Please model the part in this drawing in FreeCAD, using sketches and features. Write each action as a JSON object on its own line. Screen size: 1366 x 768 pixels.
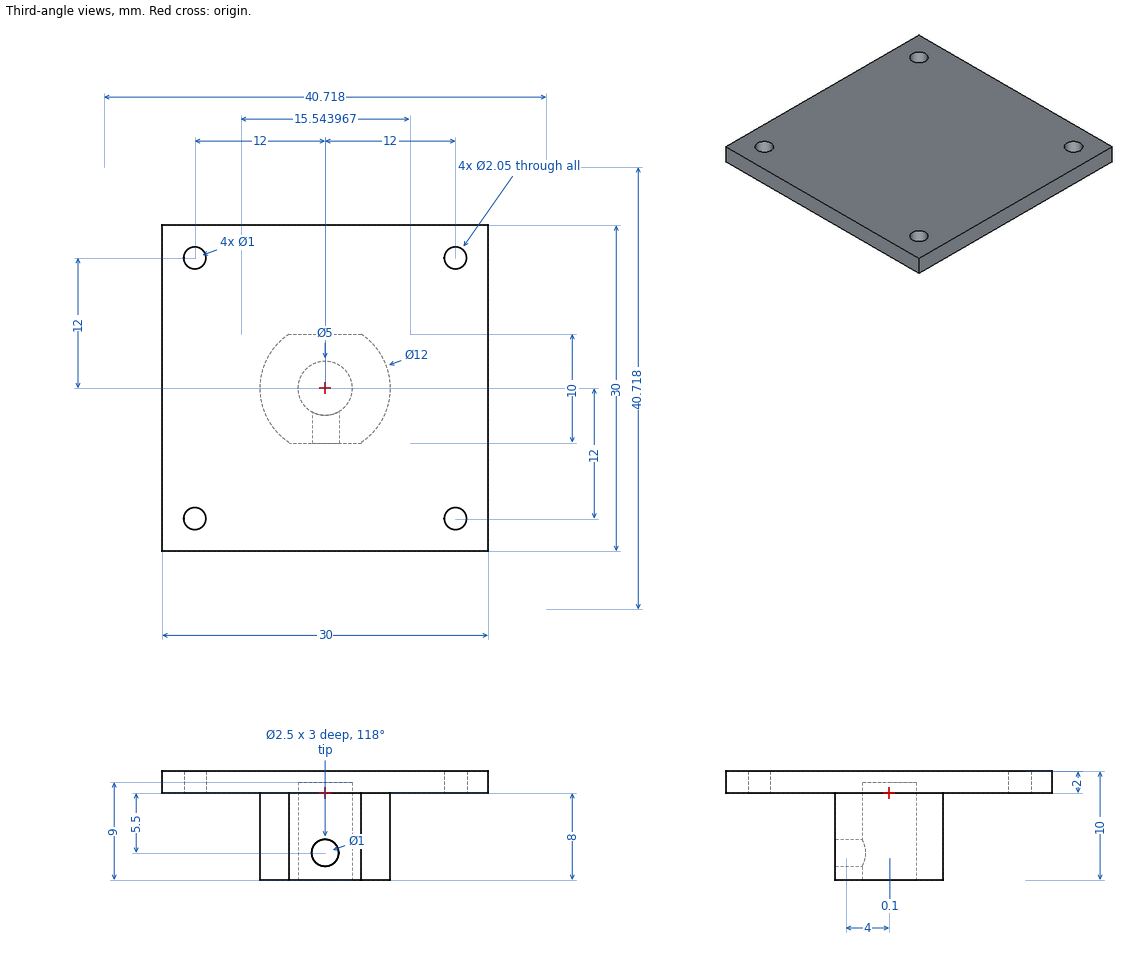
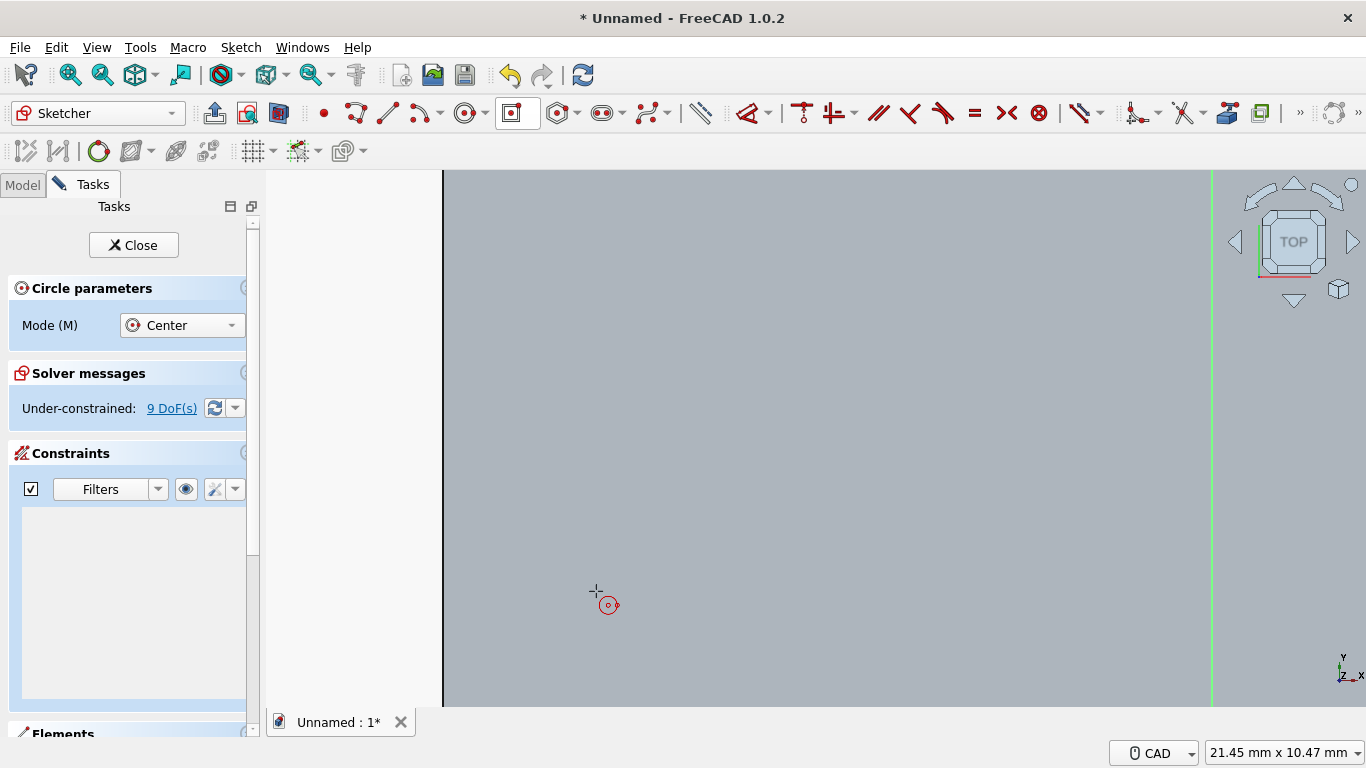
{"action": "scroll", "coordinate": [595, 591], "scroll_direction": "down", "scroll_amount": 7}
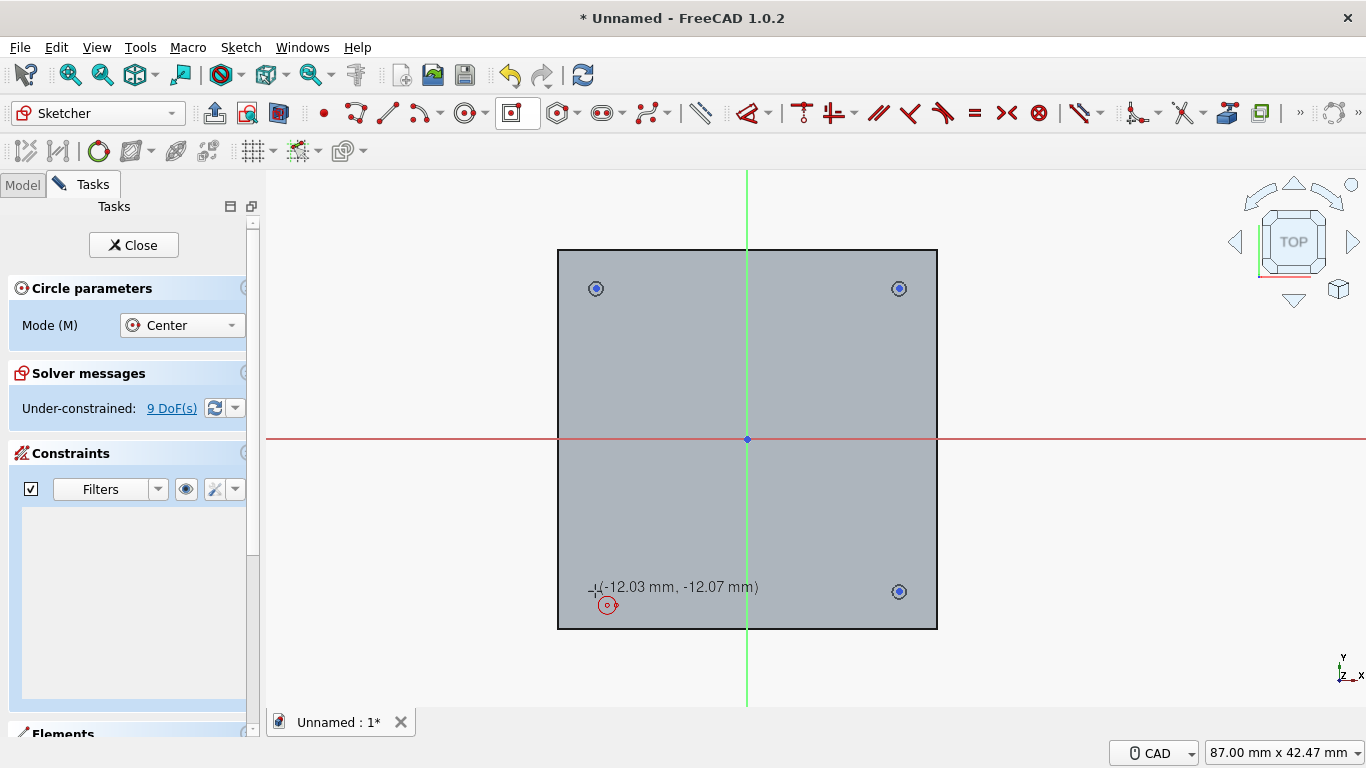
{"action": "left_click", "coordinate": [596, 591]}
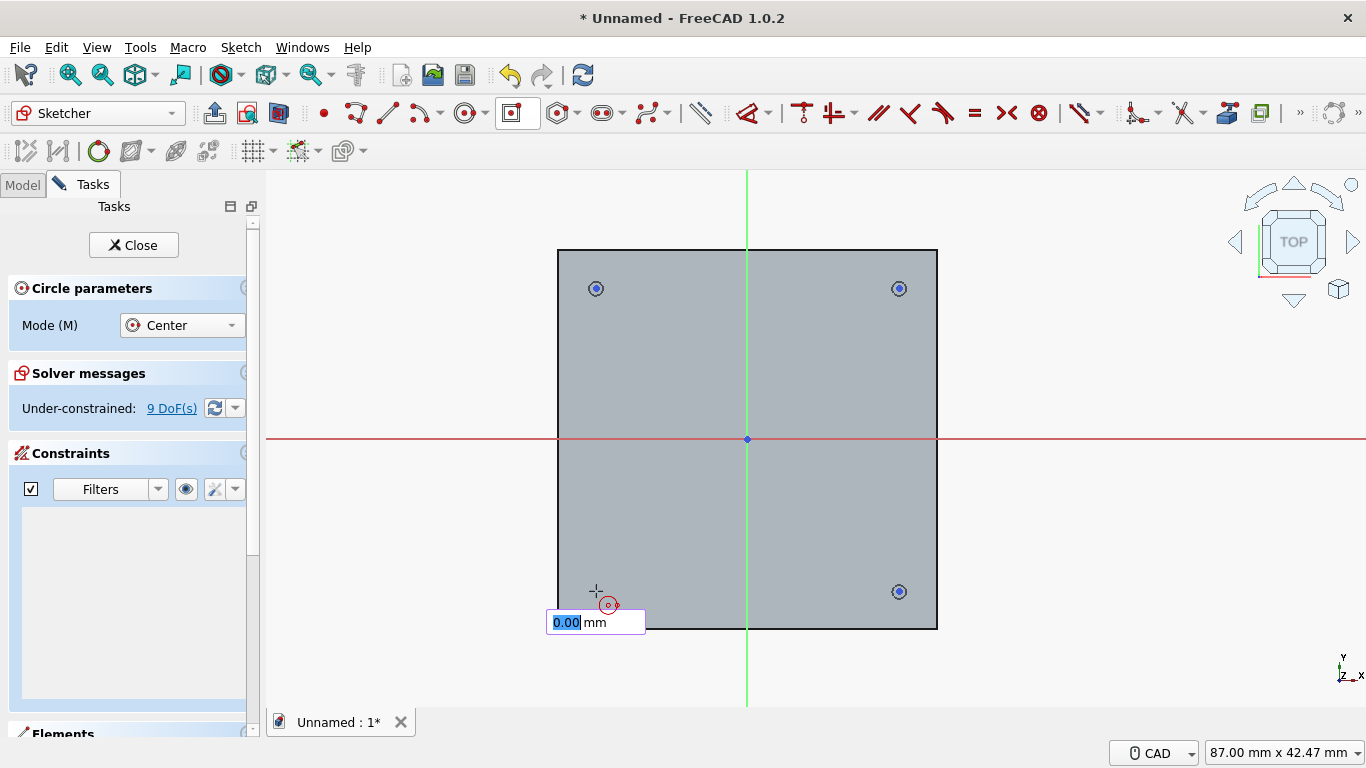
{"action": "scroll", "coordinate": [600, 587], "scroll_direction": "up", "scroll_amount": 5}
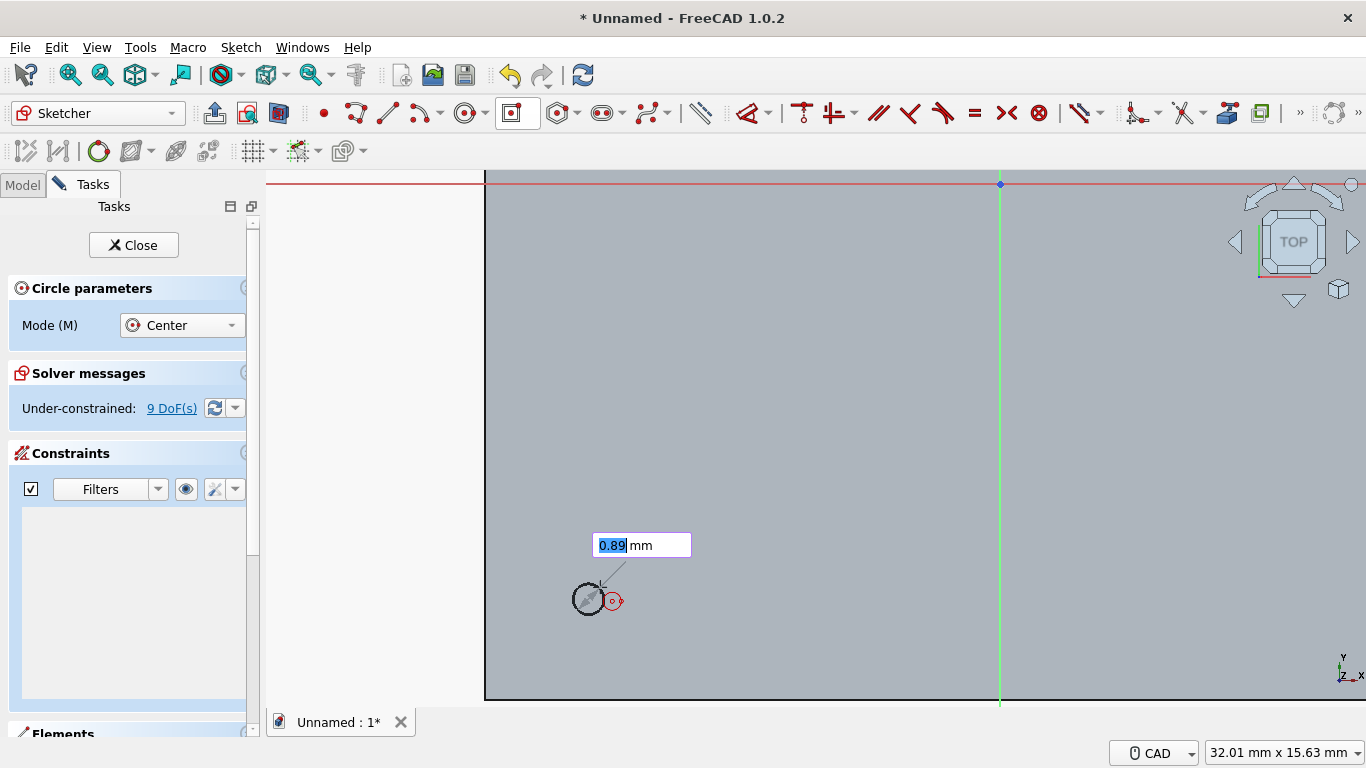
{"action": "left_click", "coordinate": [600, 584]}
{"action": "key", "text": "Escape"}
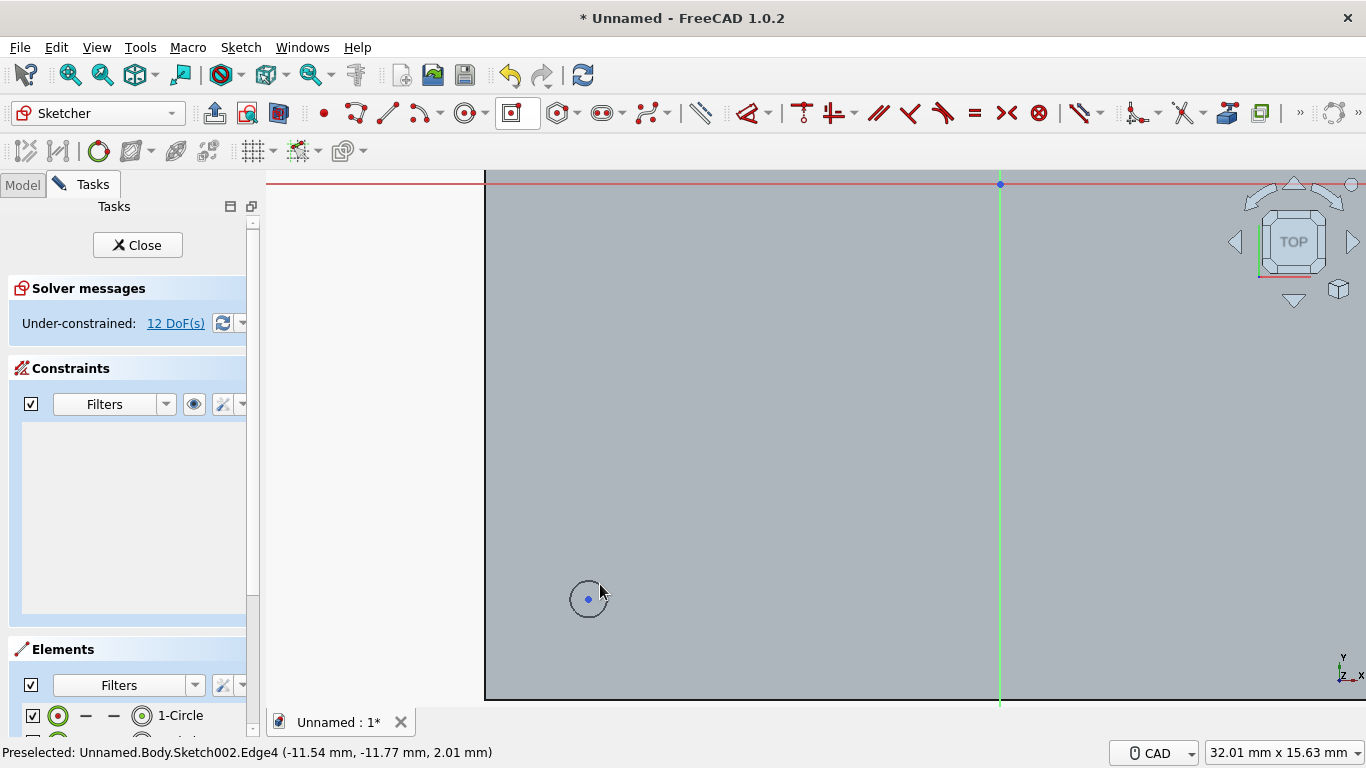
{"action": "scroll", "coordinate": [600, 587], "scroll_direction": "down", "scroll_amount": 5}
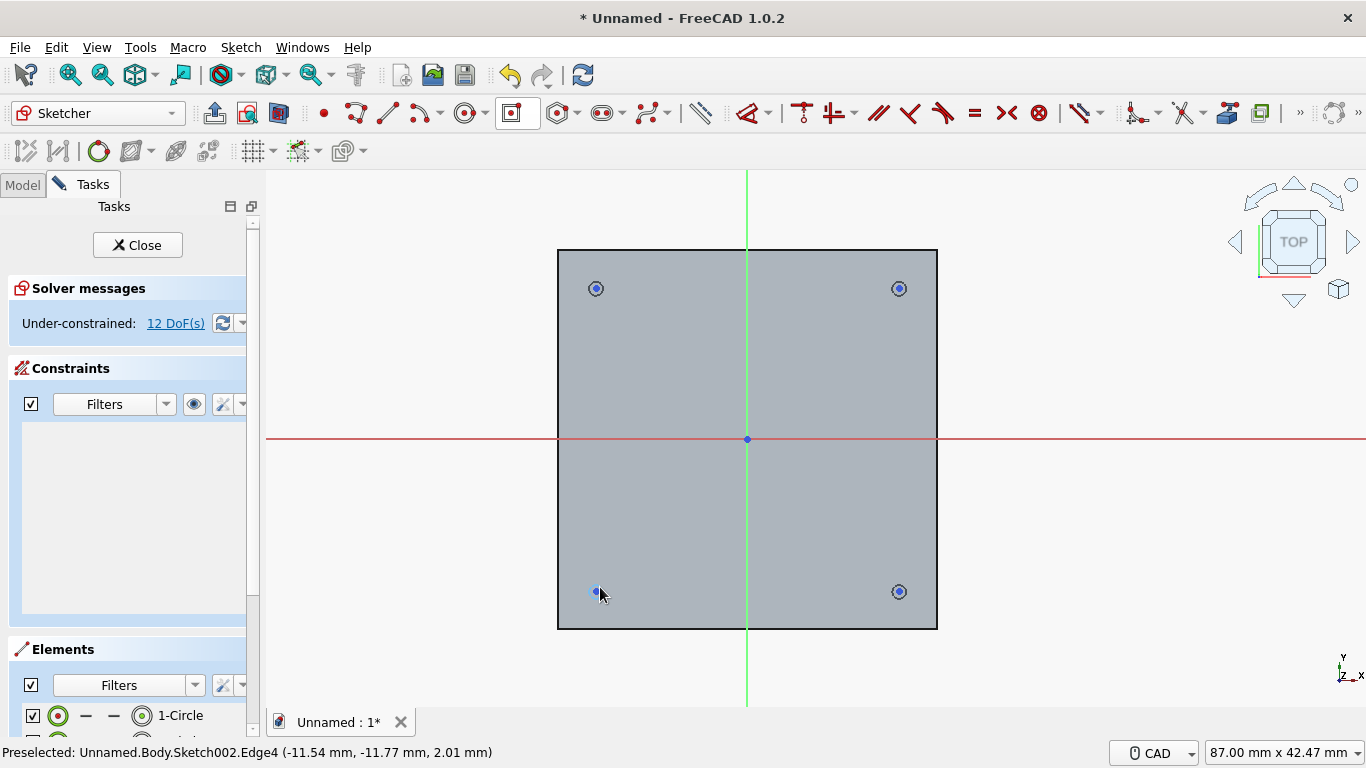
{"action": "scroll", "coordinate": [601, 284], "scroll_direction": "up", "scroll_amount": 4}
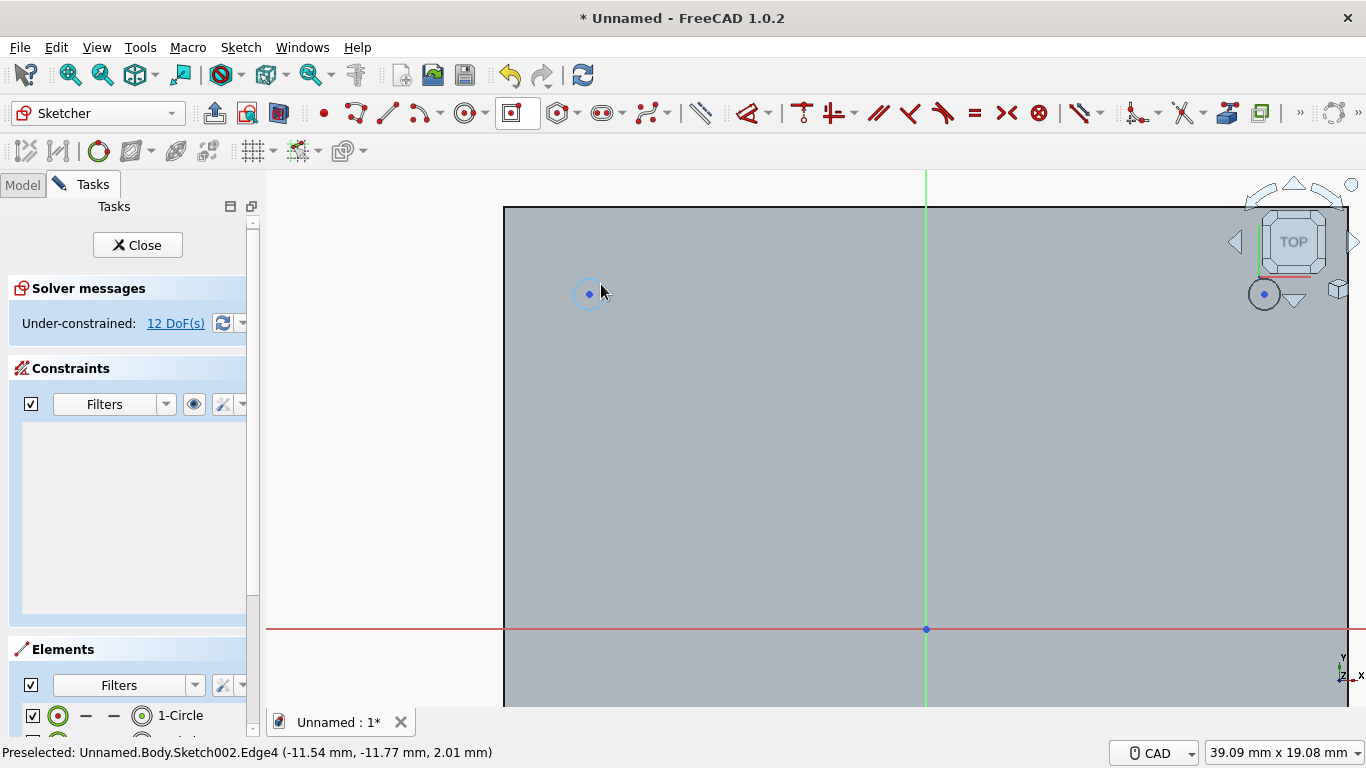
{"action": "left_click", "coordinate": [600, 283]}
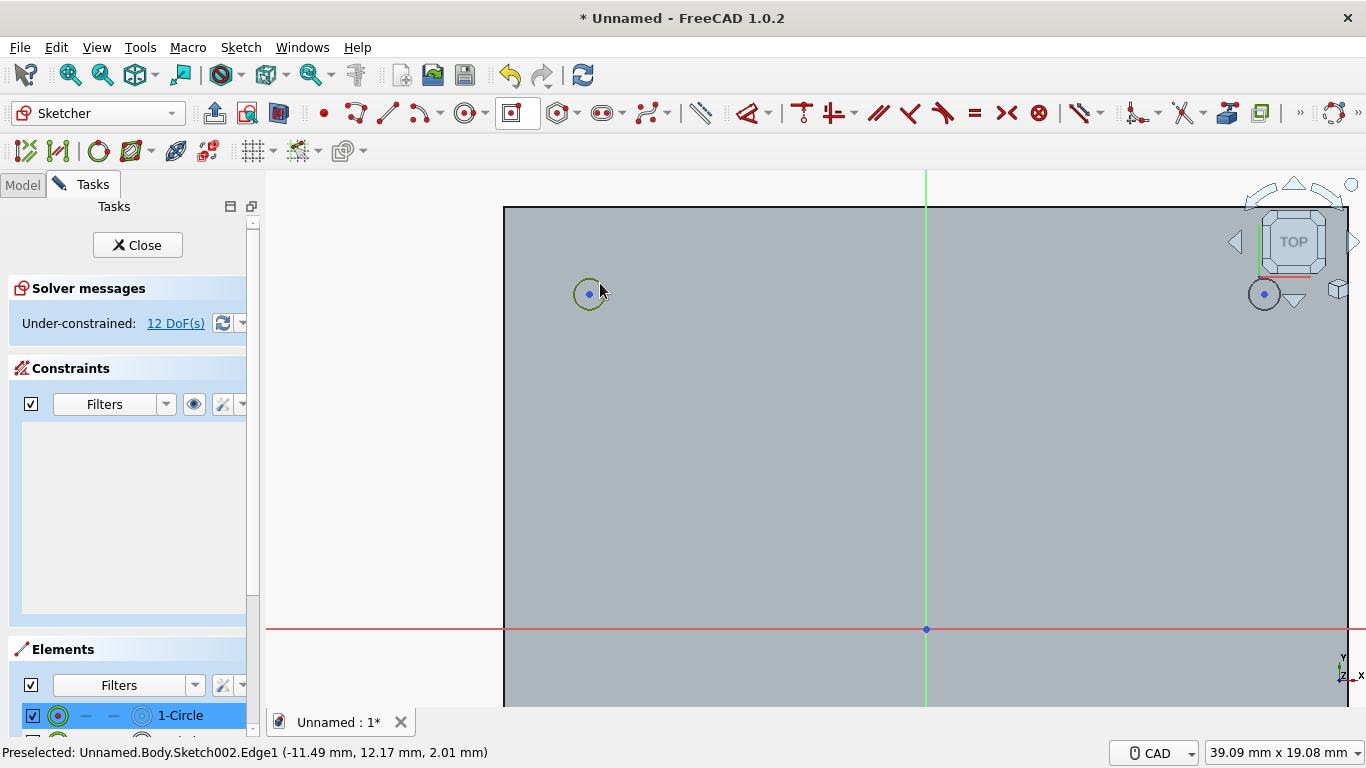
{"action": "scroll", "coordinate": [602, 283], "scroll_direction": "down", "scroll_amount": 4}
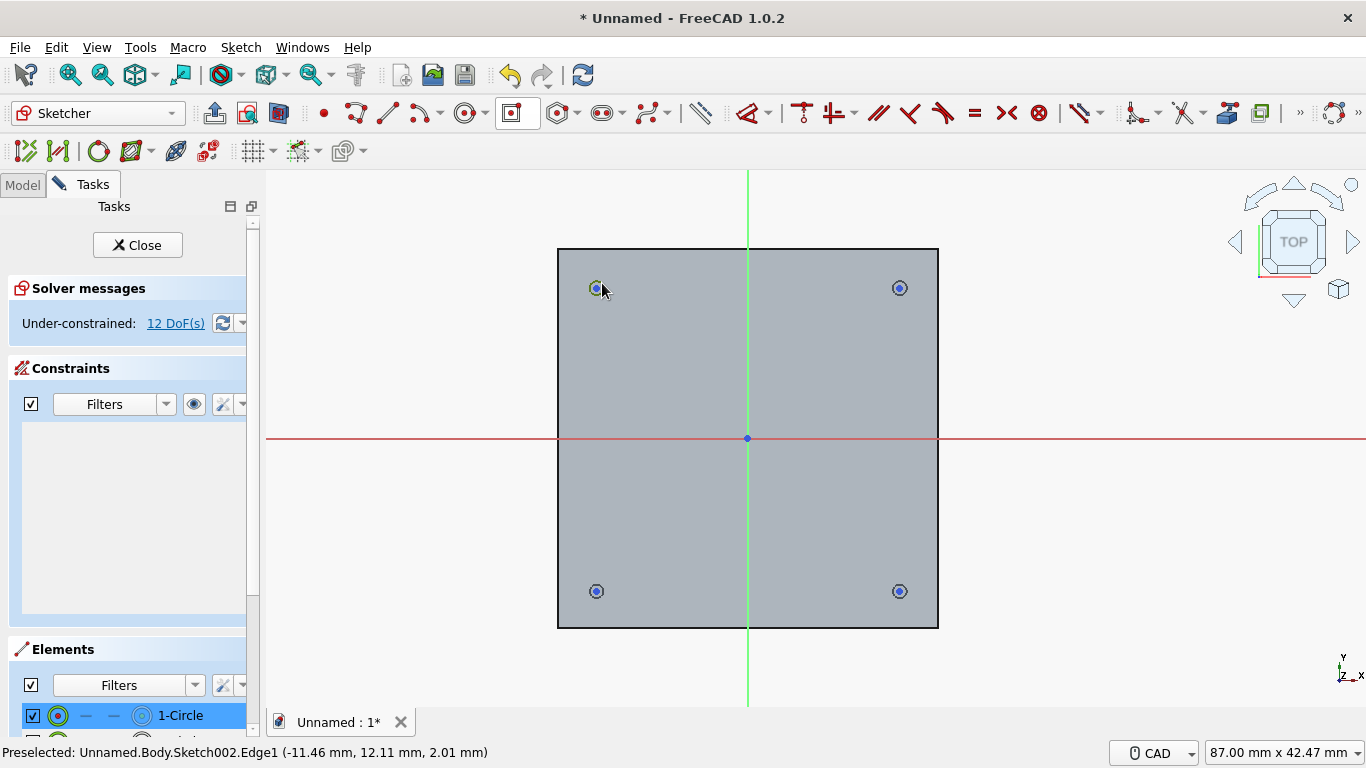
{"action": "scroll", "coordinate": [905, 283], "scroll_direction": "up", "scroll_amount": 4}